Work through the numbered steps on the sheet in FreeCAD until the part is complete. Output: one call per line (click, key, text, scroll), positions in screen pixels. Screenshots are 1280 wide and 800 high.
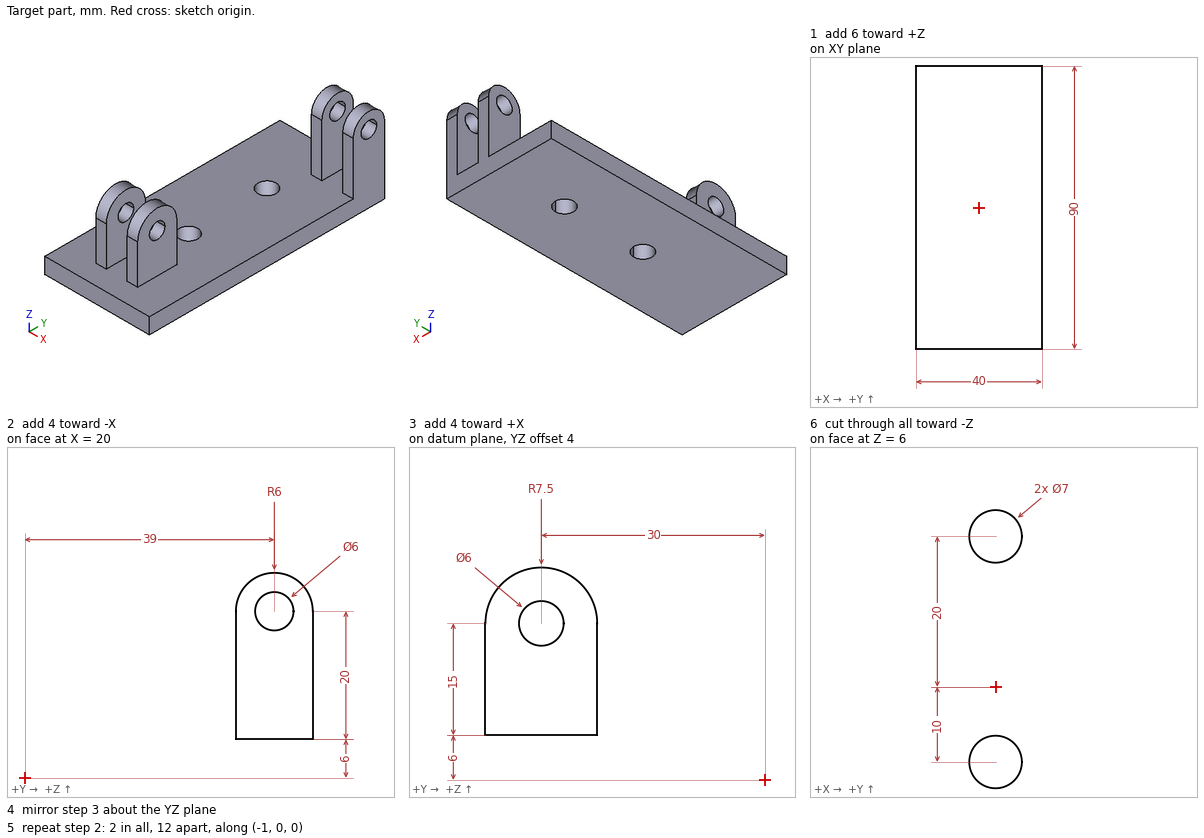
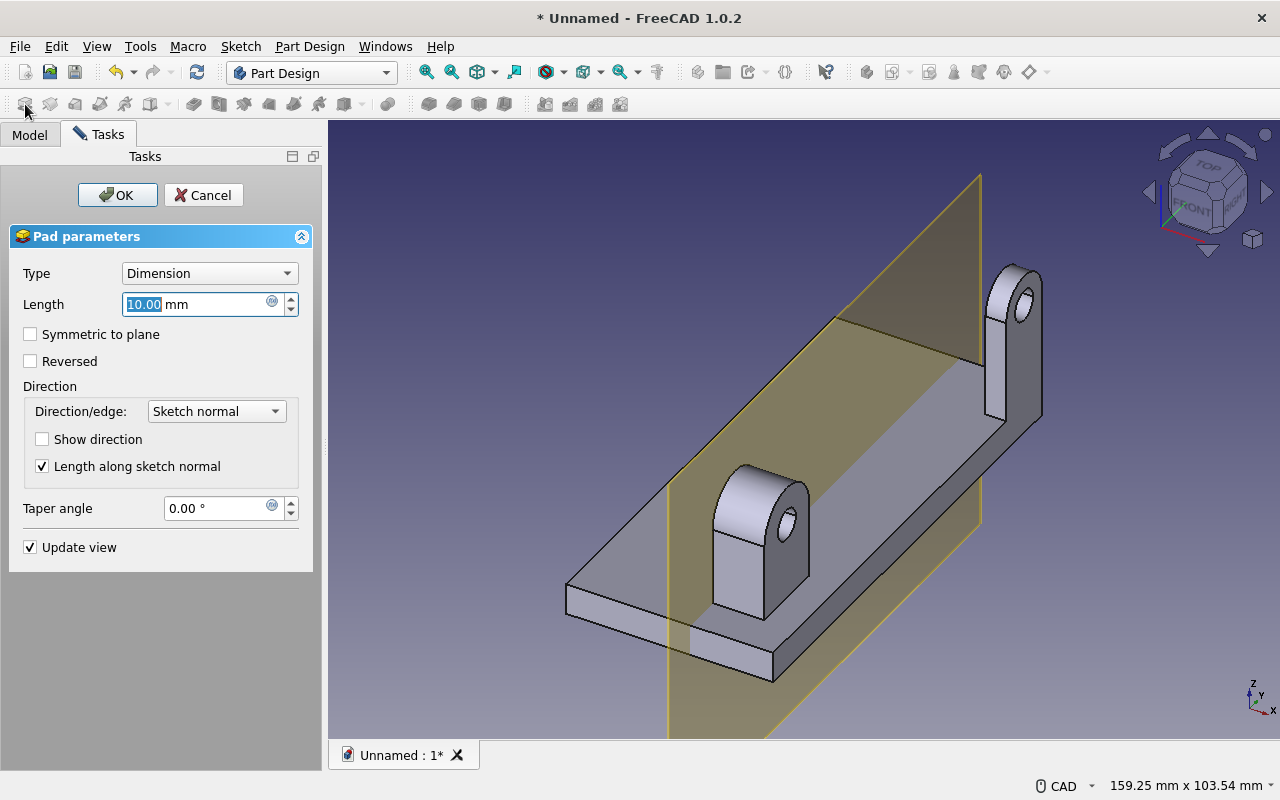
text(4)
key(Tab)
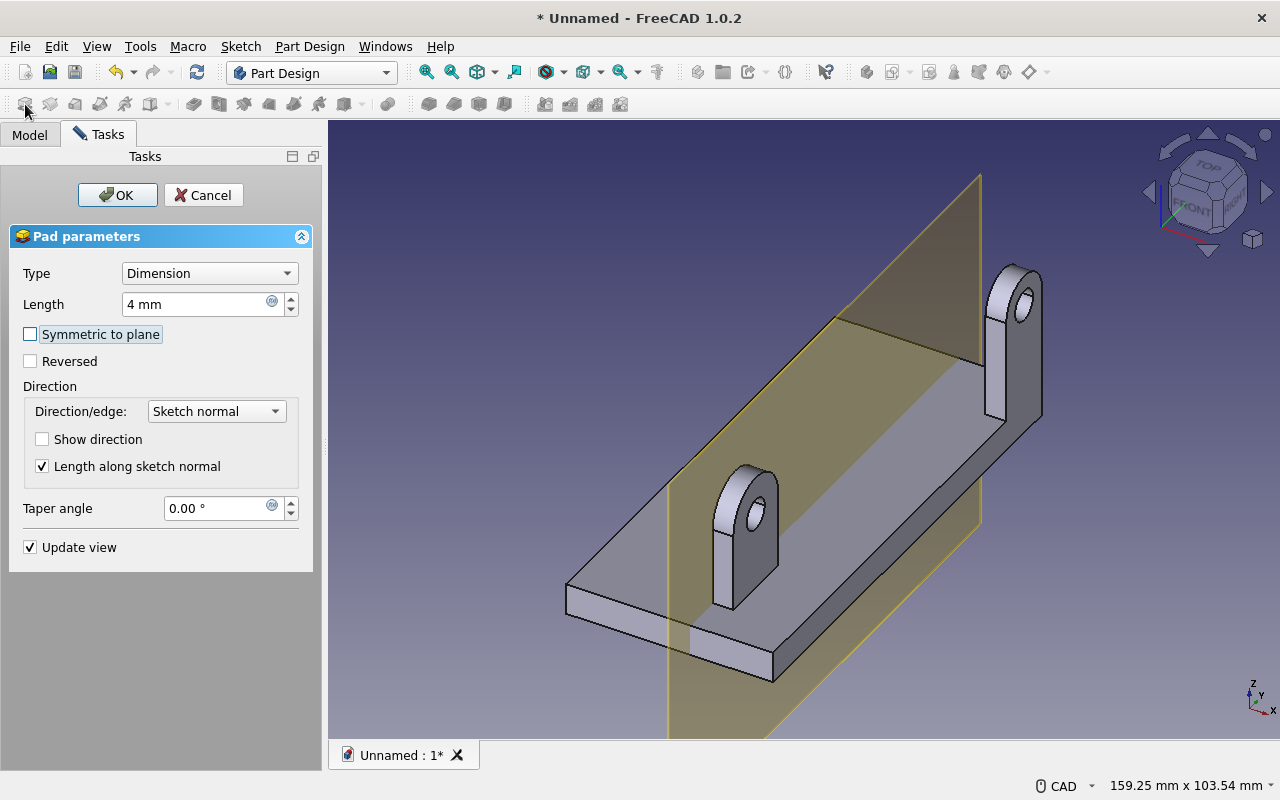
click(118, 195)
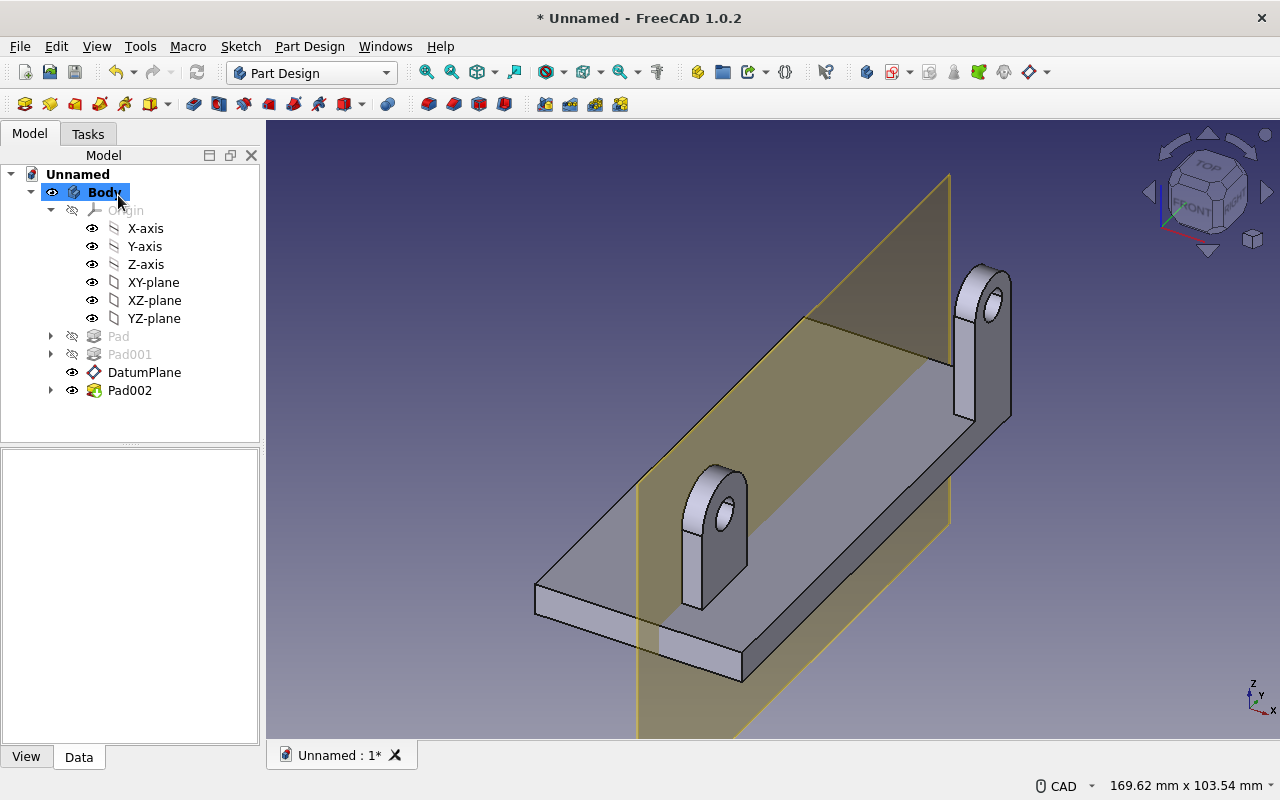
click(117, 372)
key(space)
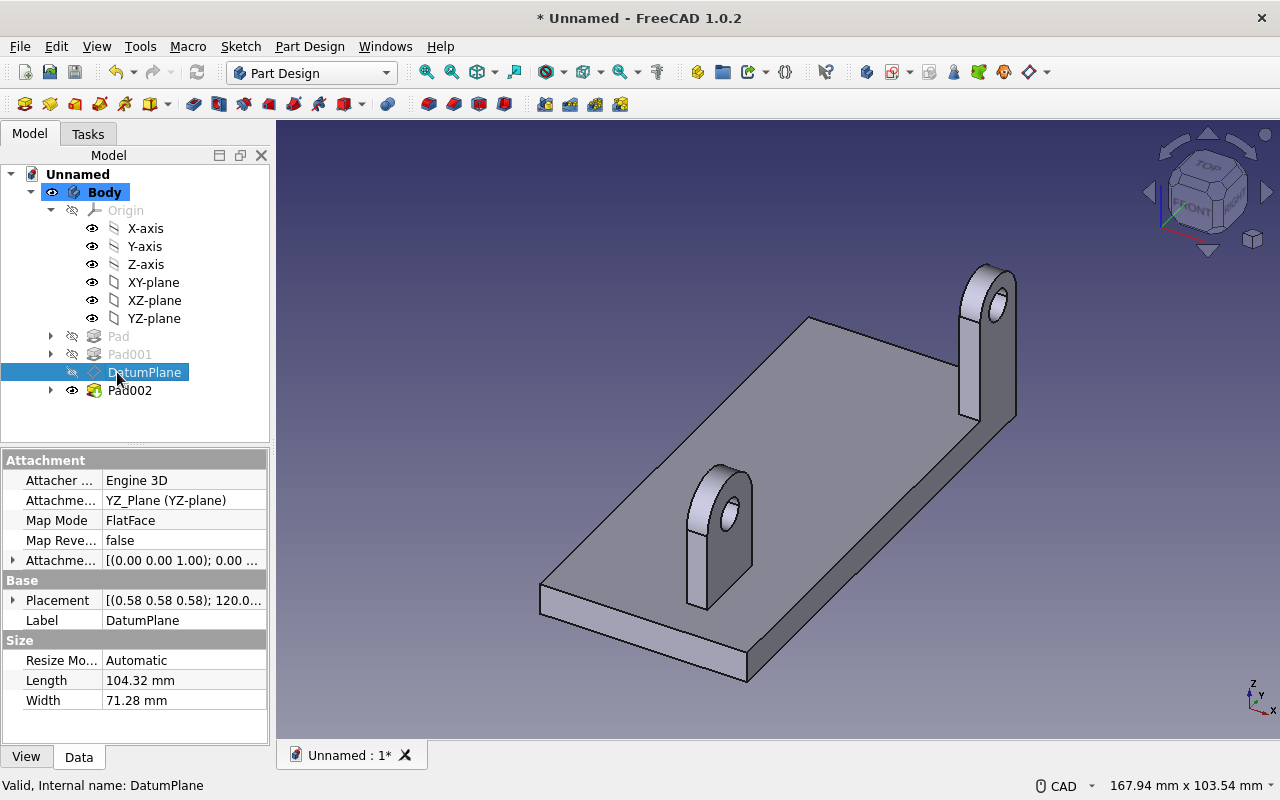
click(117, 390)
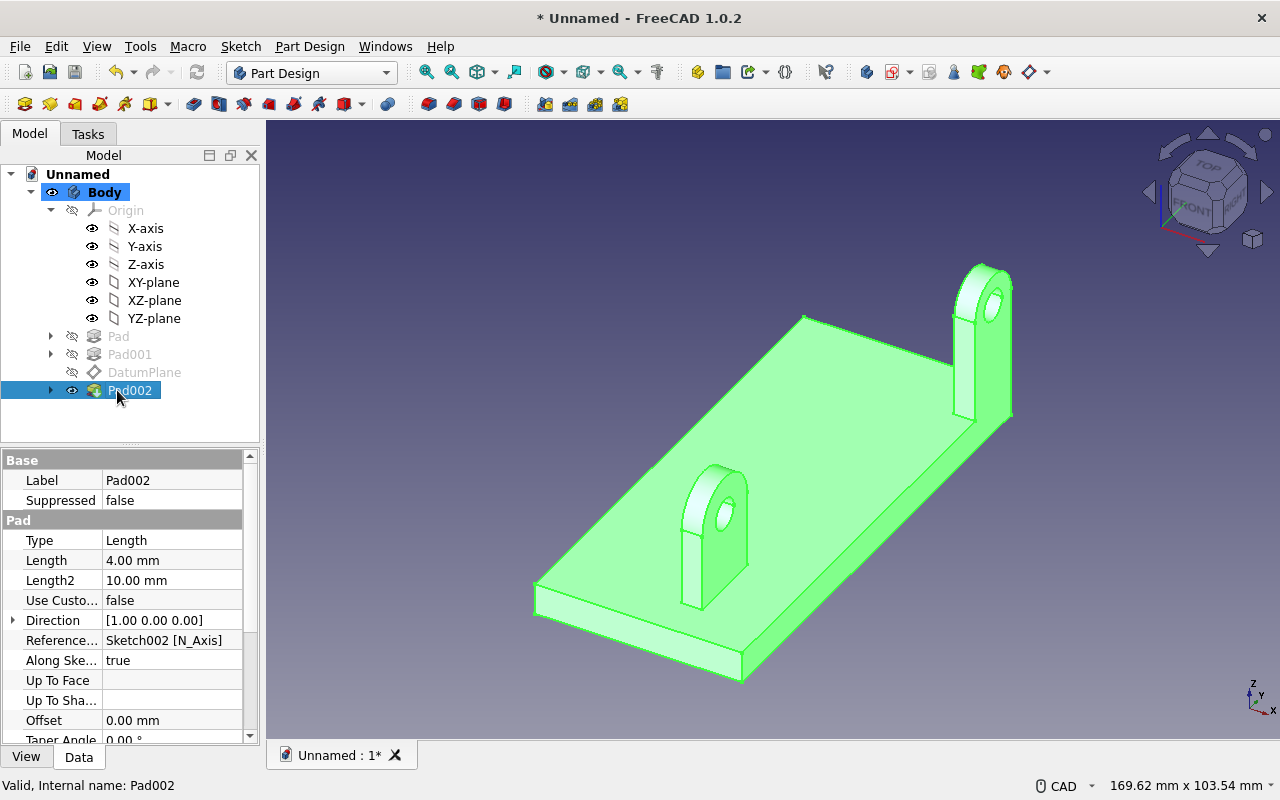
click(545, 104)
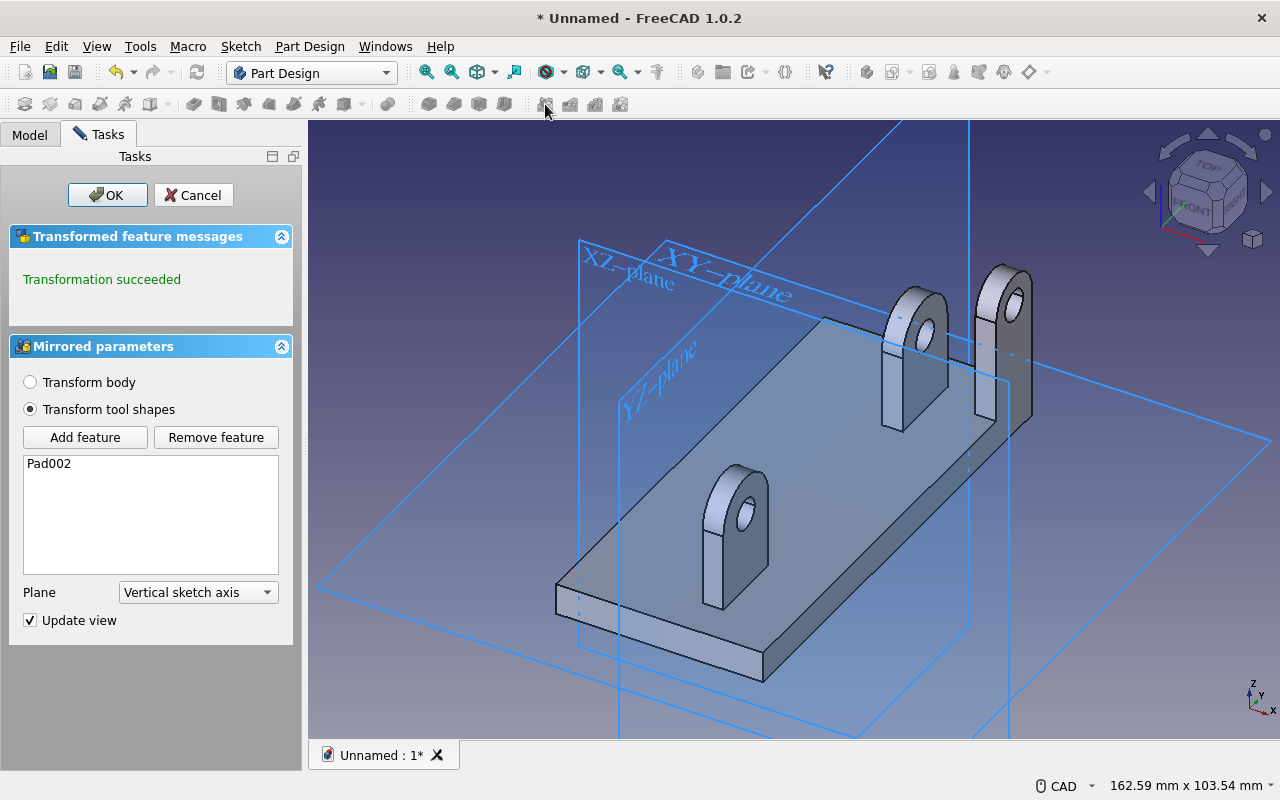
click(199, 592)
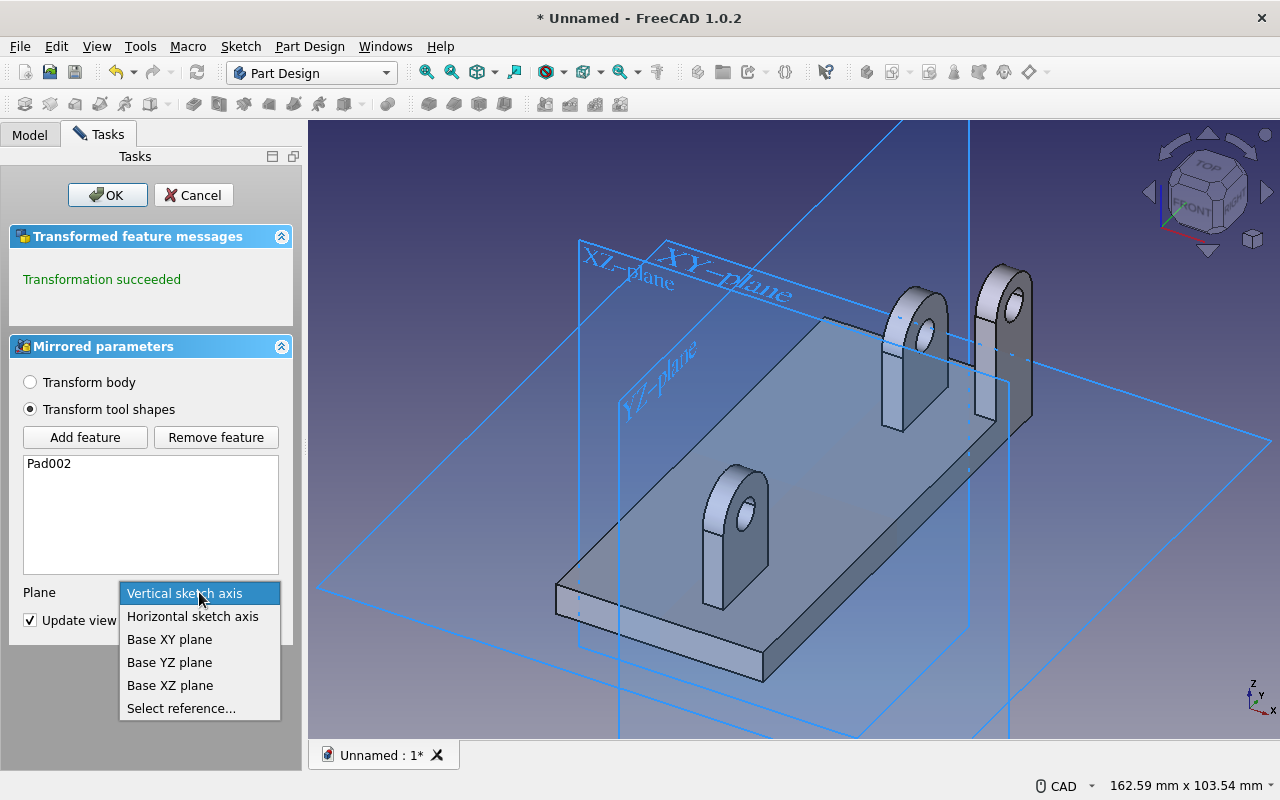
click(198, 662)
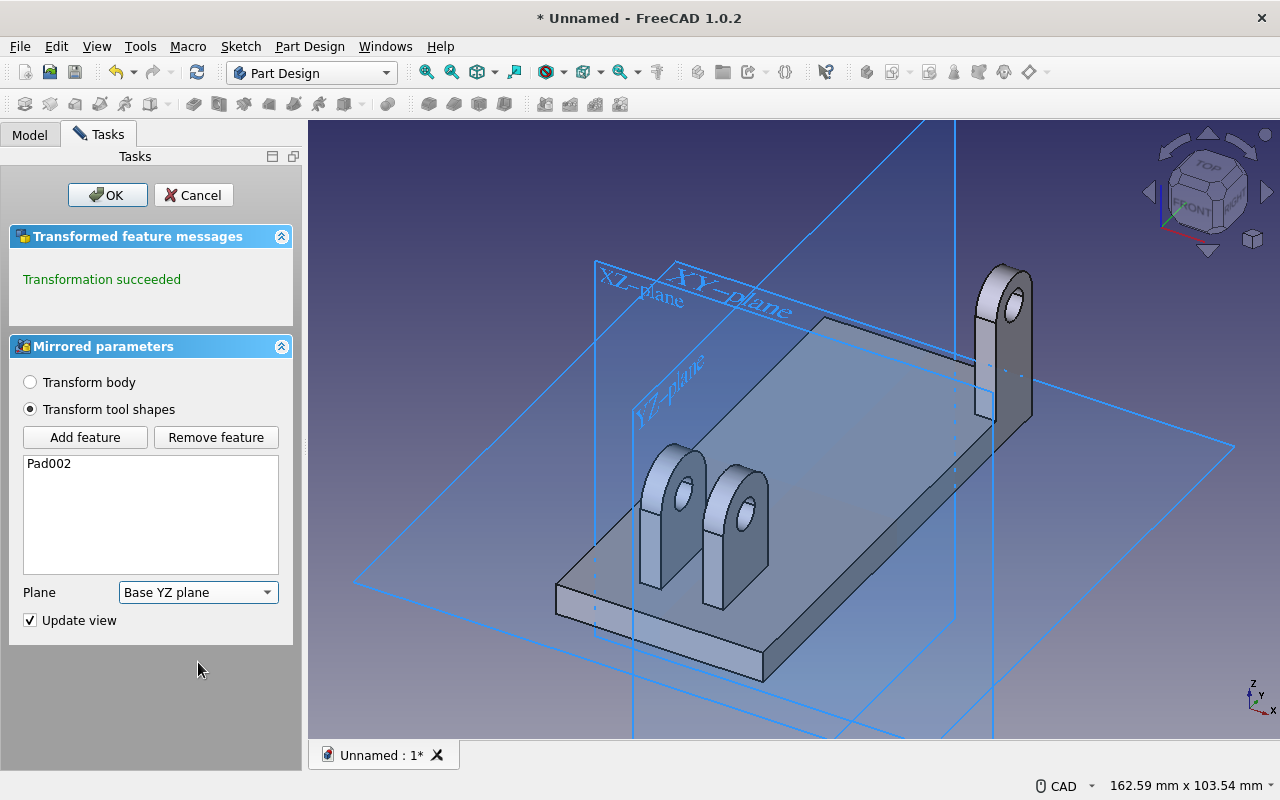
click(108, 195)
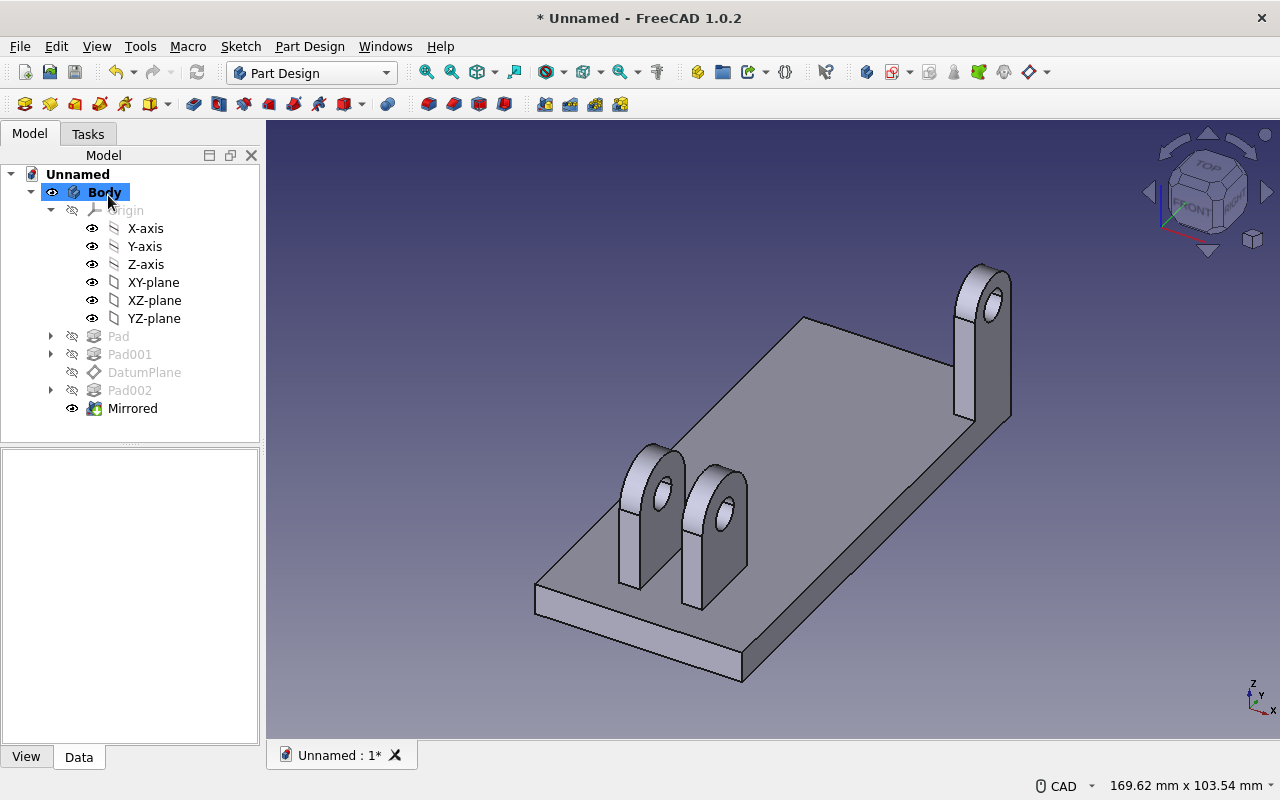
click(117, 354)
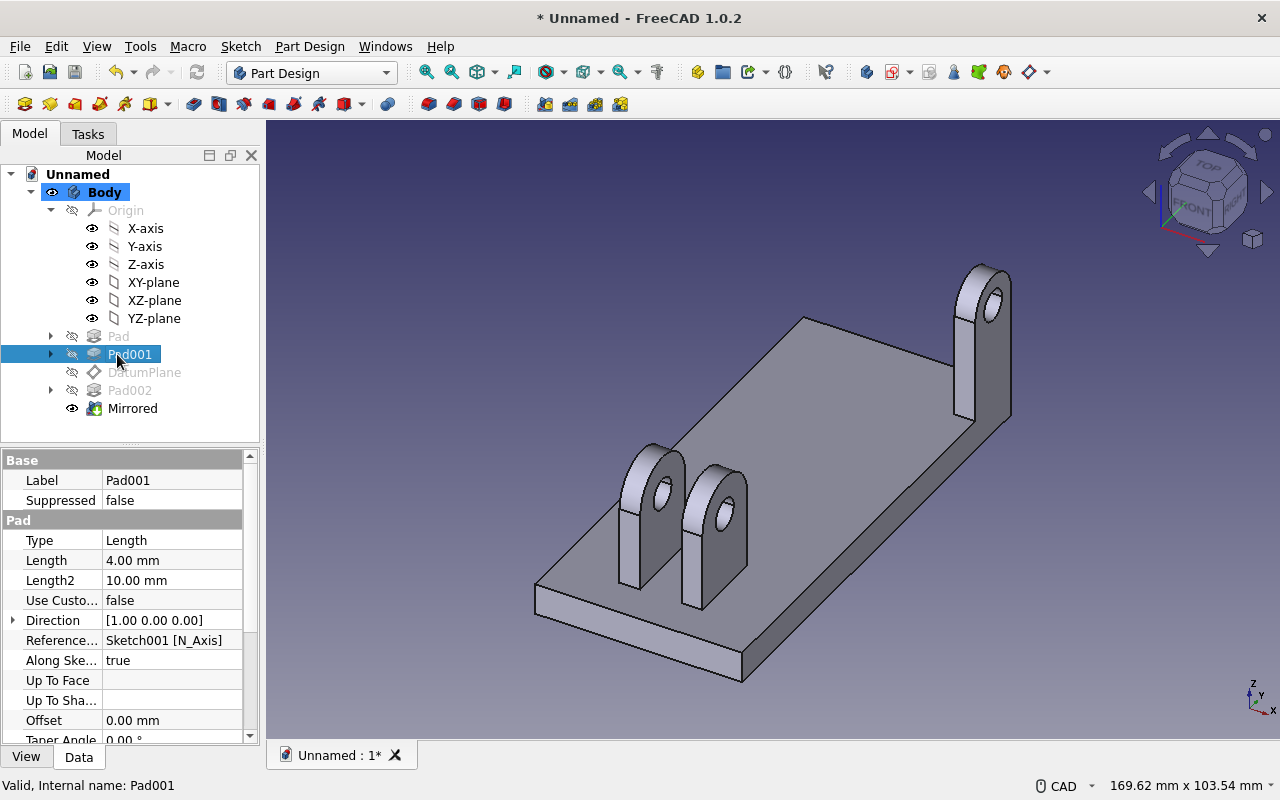
click(570, 104)